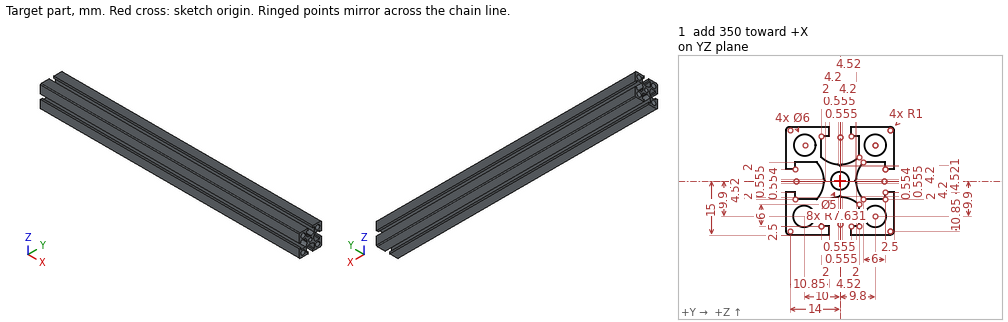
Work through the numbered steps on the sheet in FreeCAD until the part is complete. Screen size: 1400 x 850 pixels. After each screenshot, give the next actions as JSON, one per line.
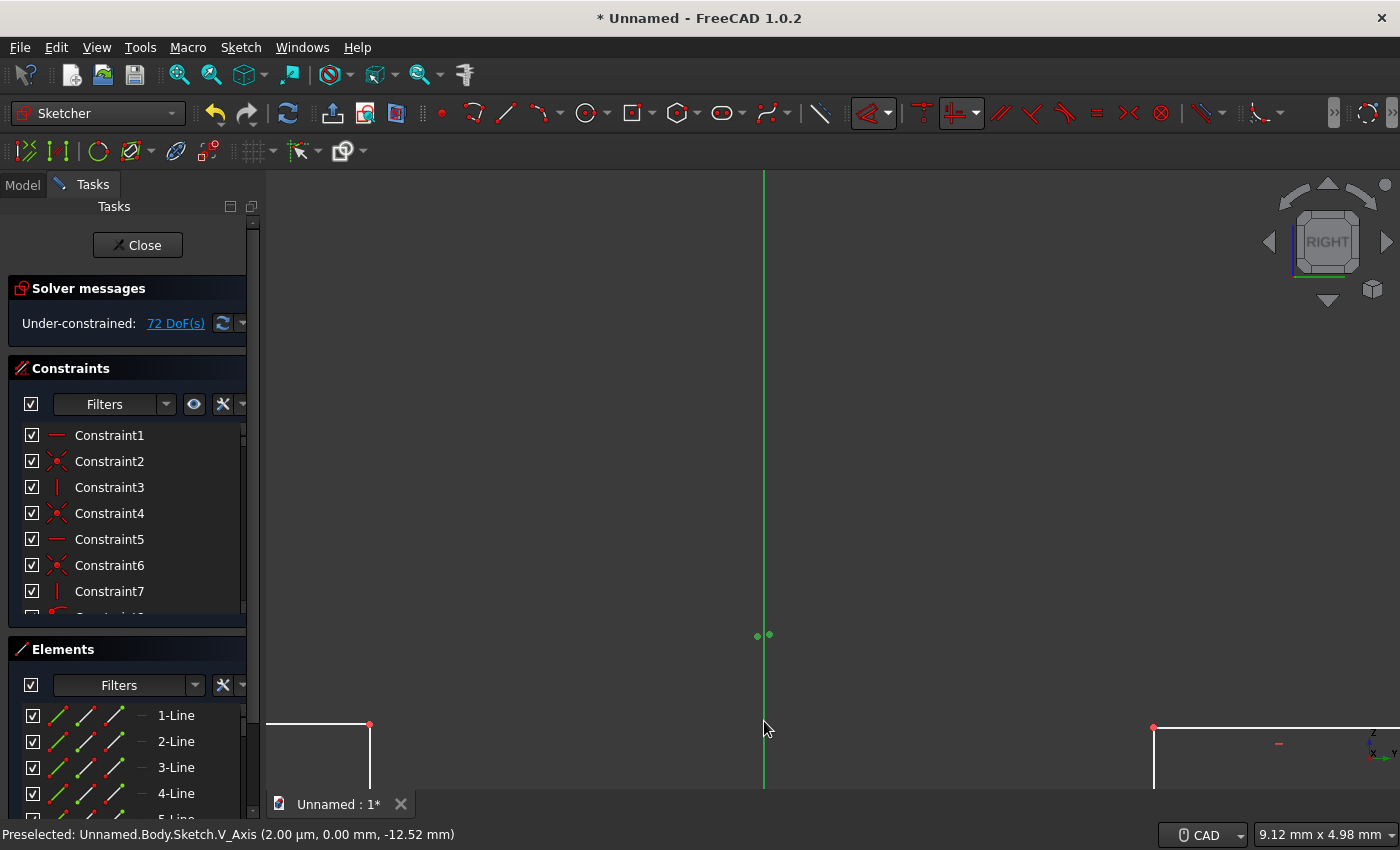
{"action": "left_click", "coordinate": [1130, 114]}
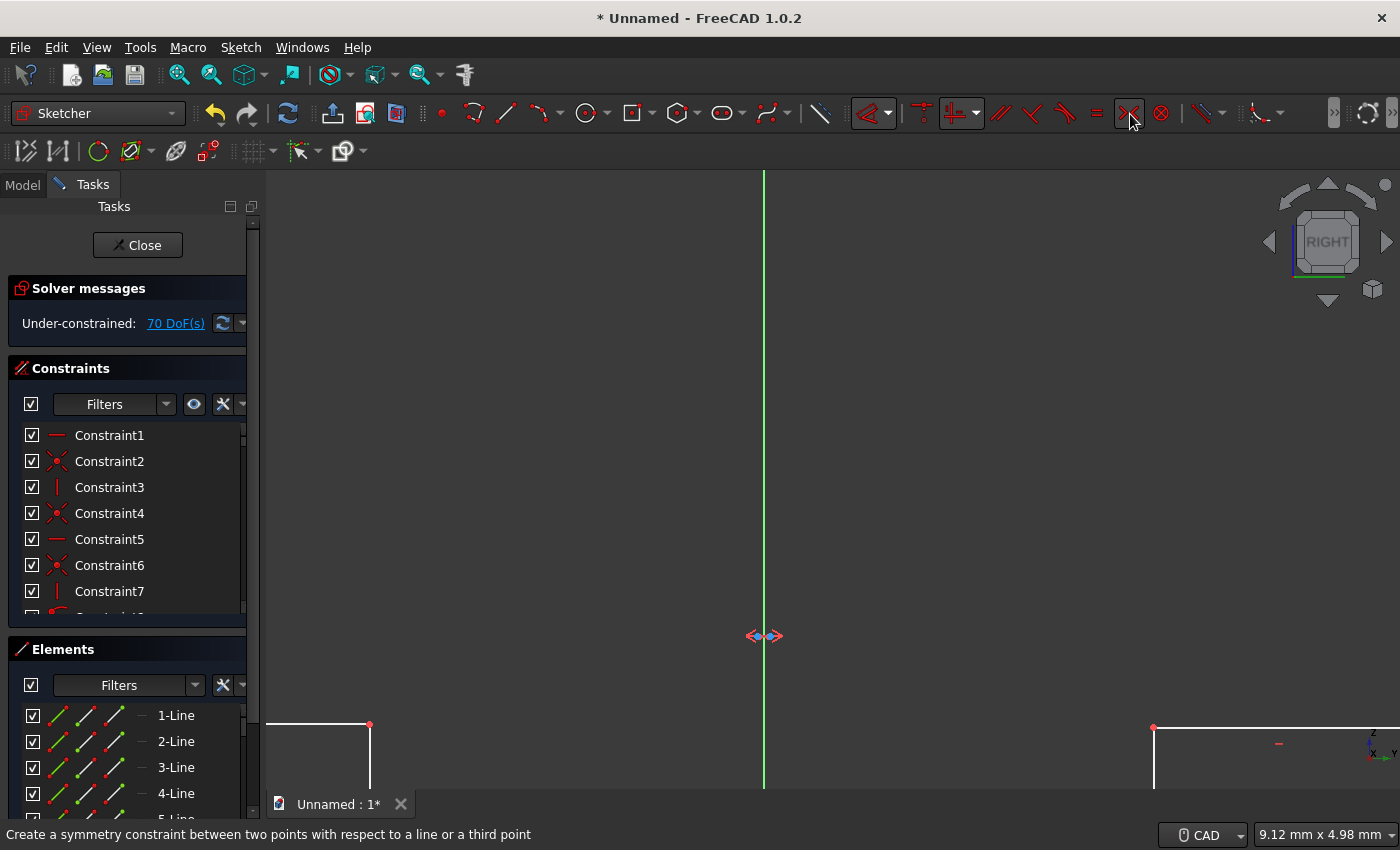
{"action": "scroll", "coordinate": [765, 643], "scroll_direction": "down", "scroll_amount": 11}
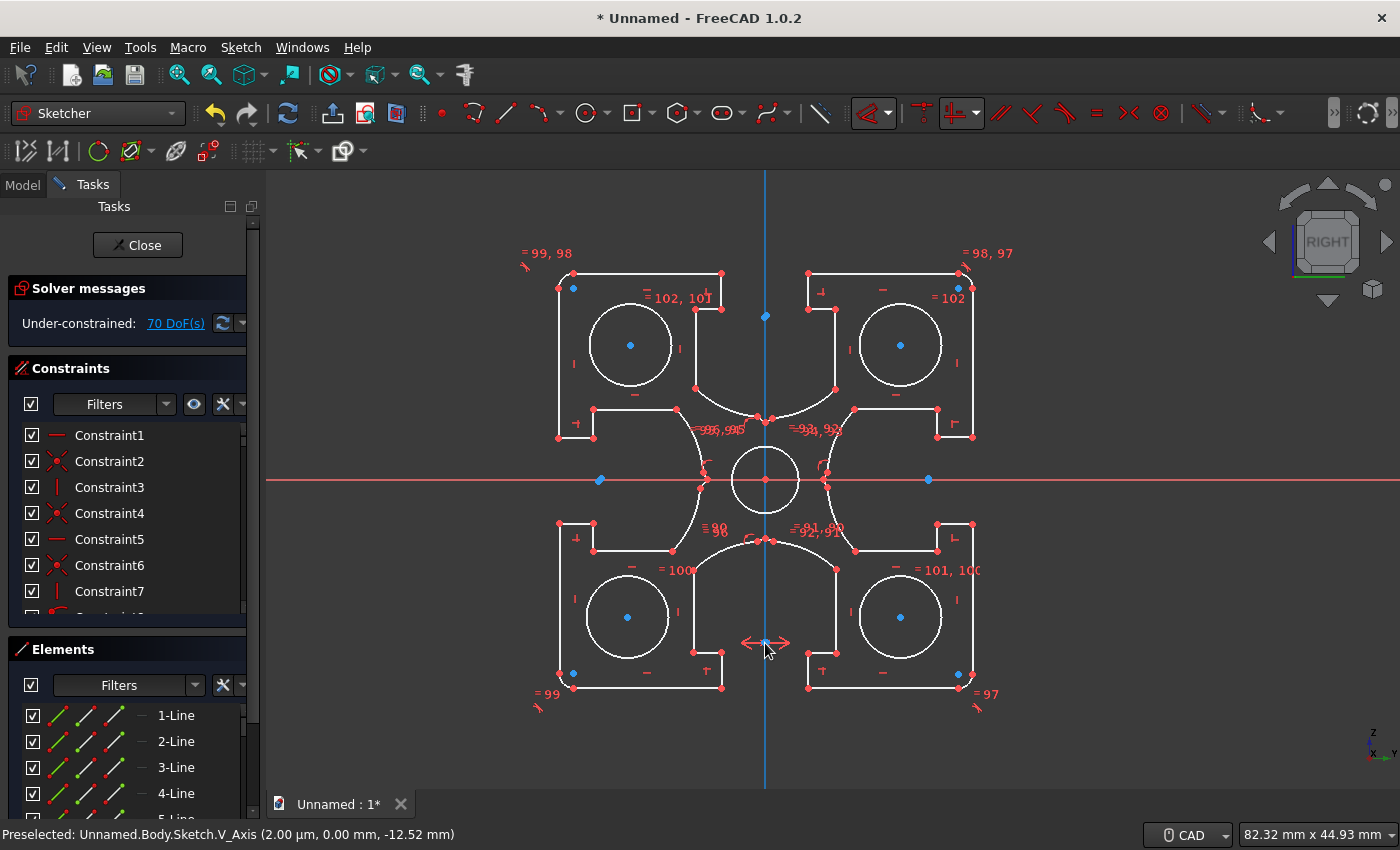
{"action": "left_click", "coordinate": [958, 674]}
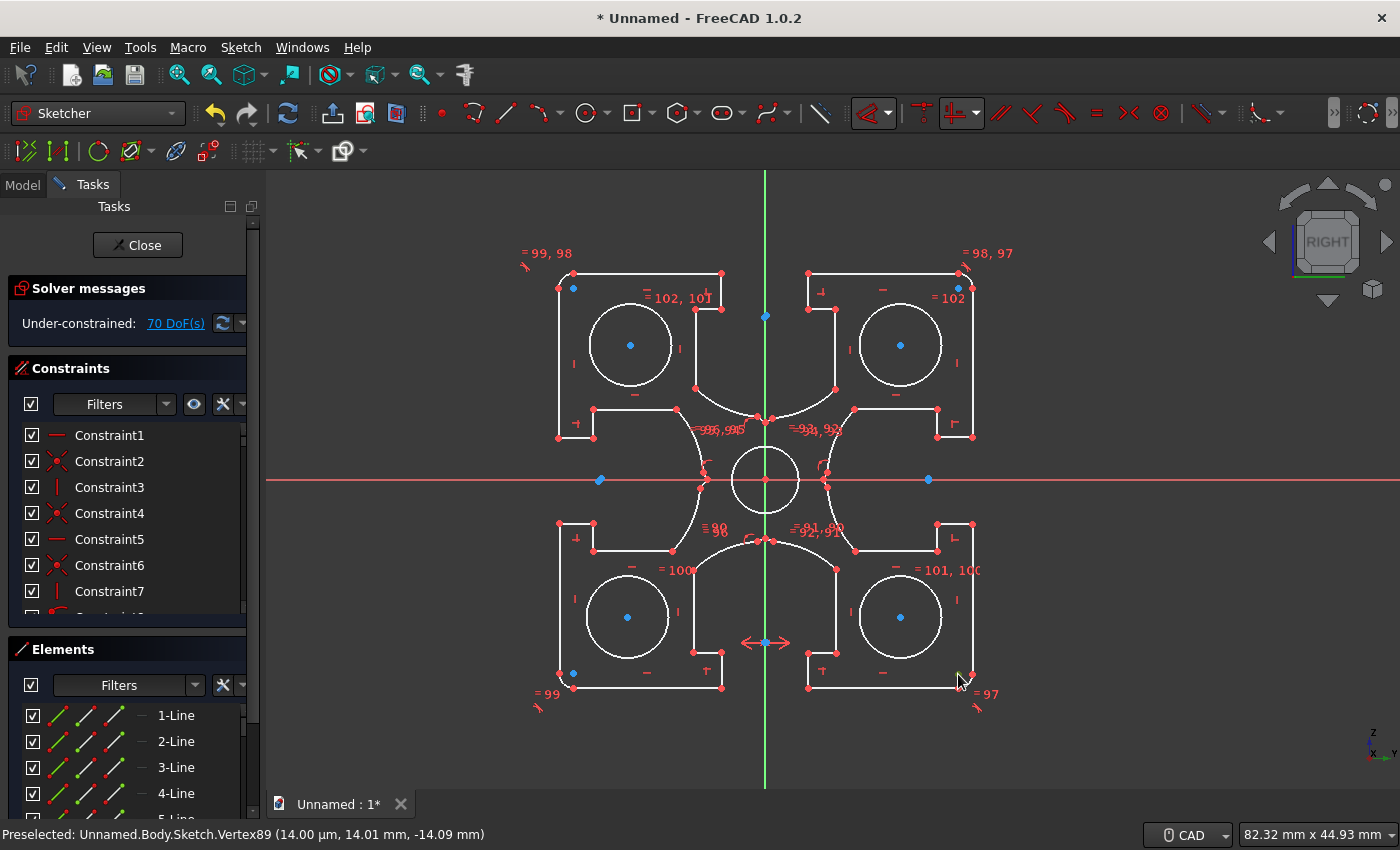
{"action": "left_click", "coordinate": [958, 288]}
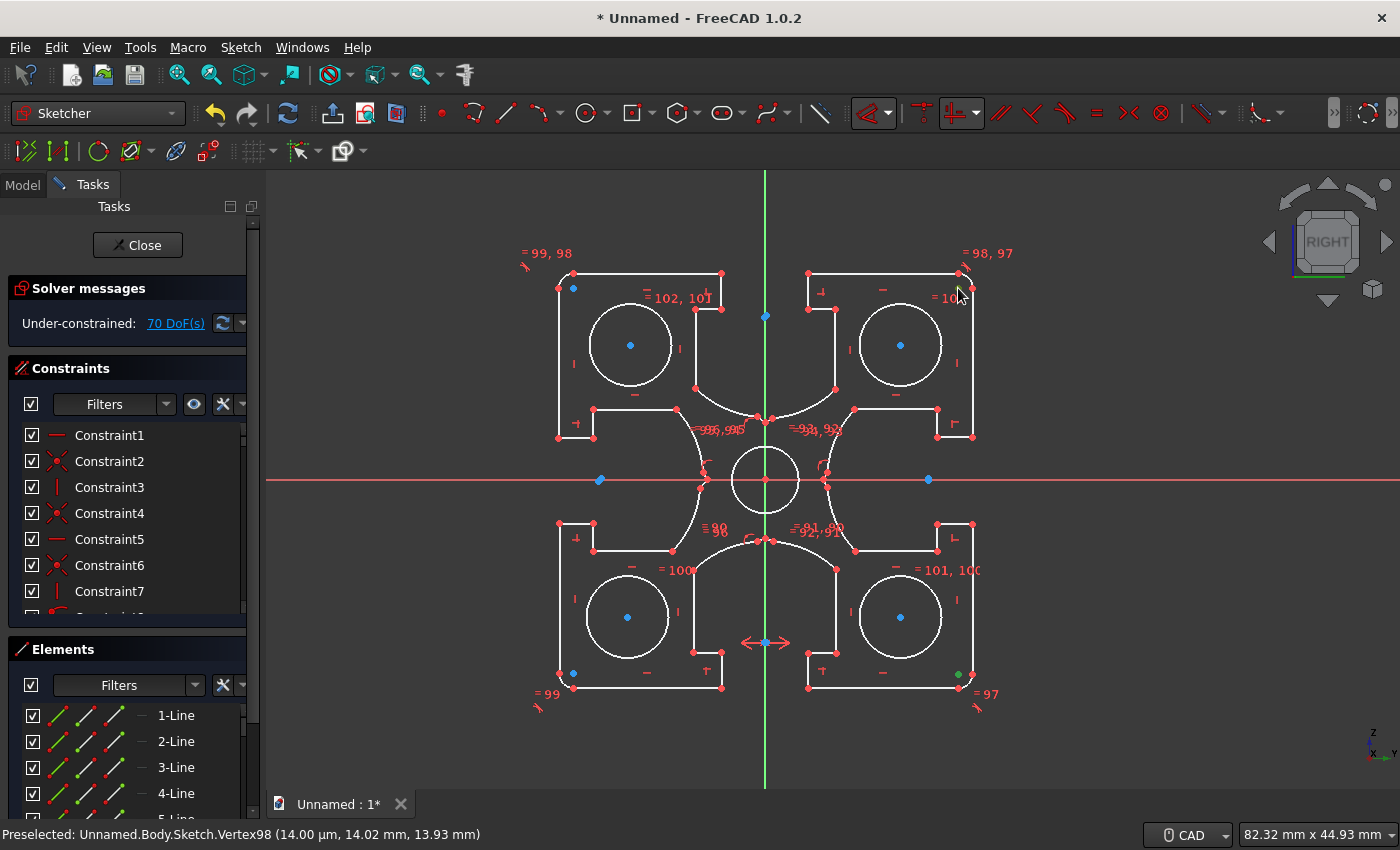
{"action": "left_click", "coordinate": [361, 480]}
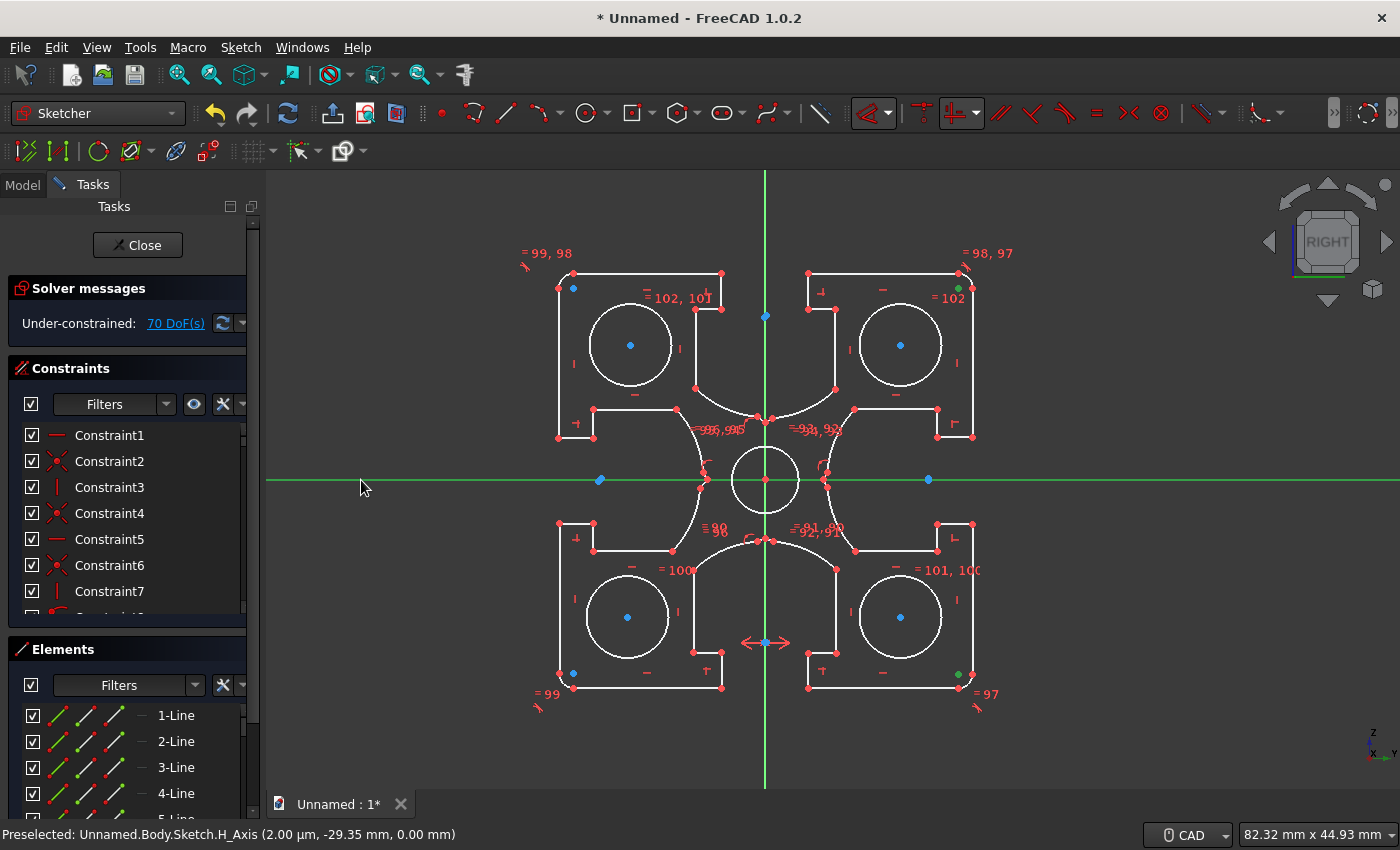
{"action": "key", "text": "s"}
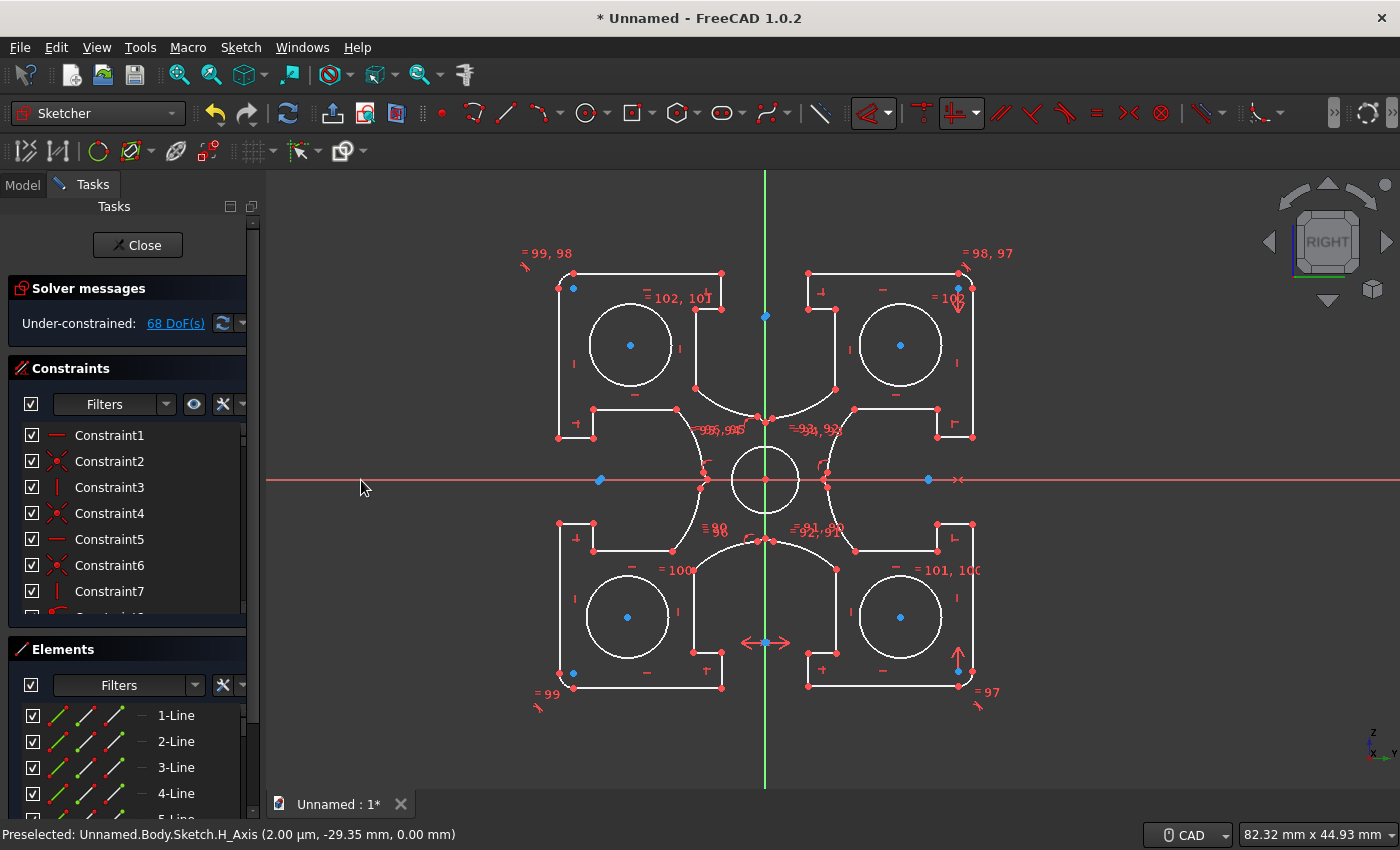
{"action": "scroll", "coordinate": [764, 317], "scroll_direction": "up", "scroll_amount": 9}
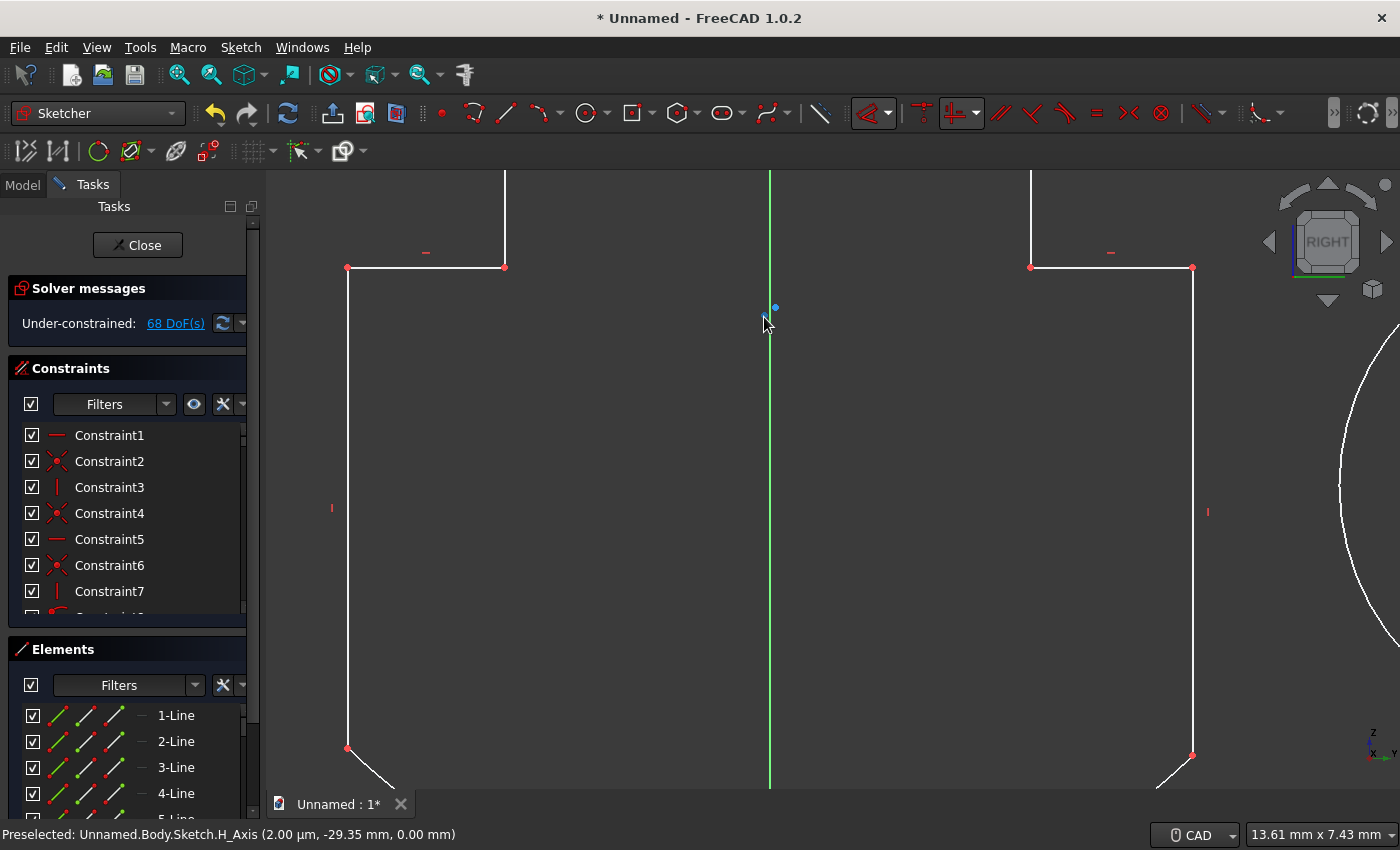
{"action": "left_click", "coordinate": [764, 316]}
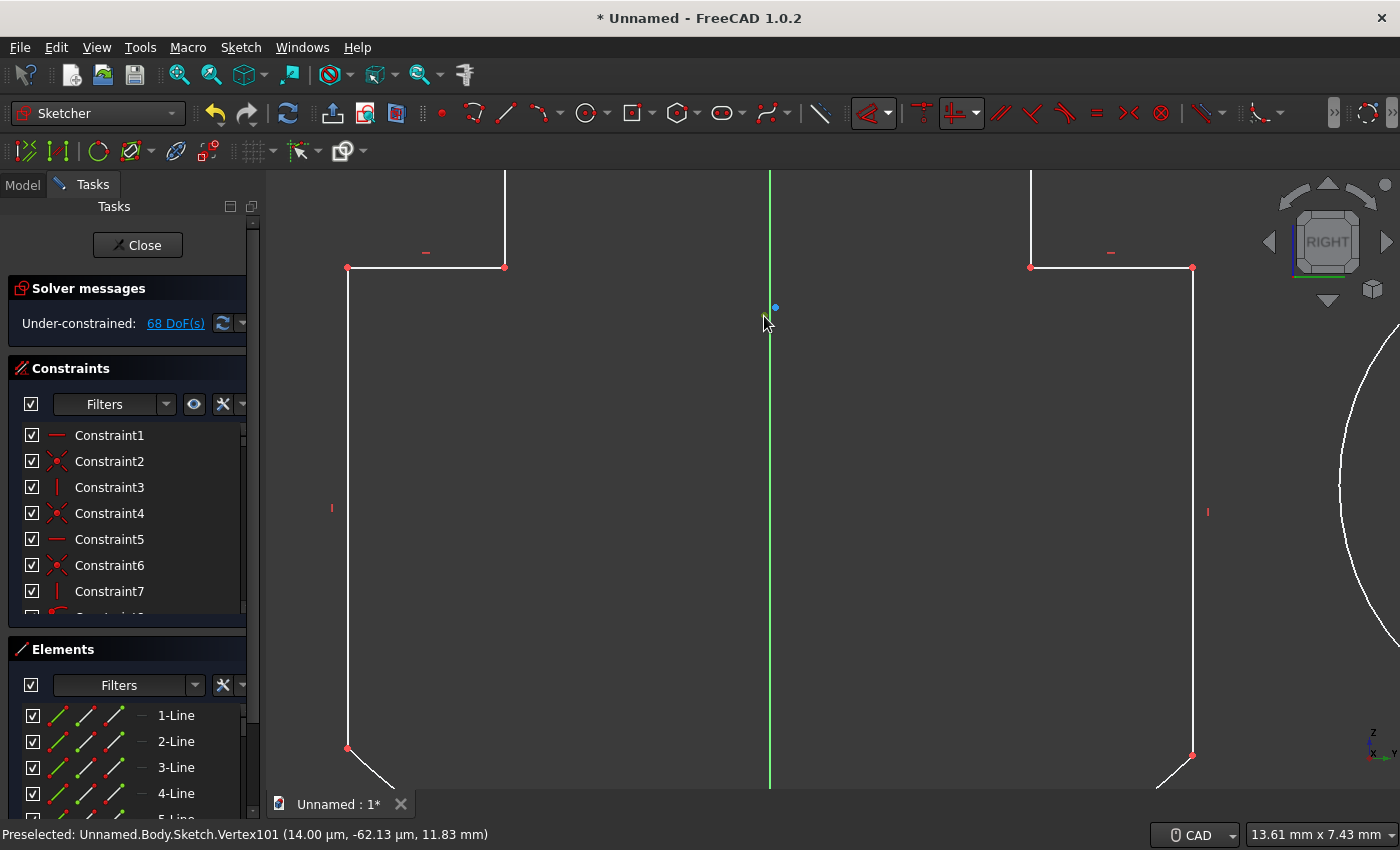
{"action": "left_click", "coordinate": [776, 308]}